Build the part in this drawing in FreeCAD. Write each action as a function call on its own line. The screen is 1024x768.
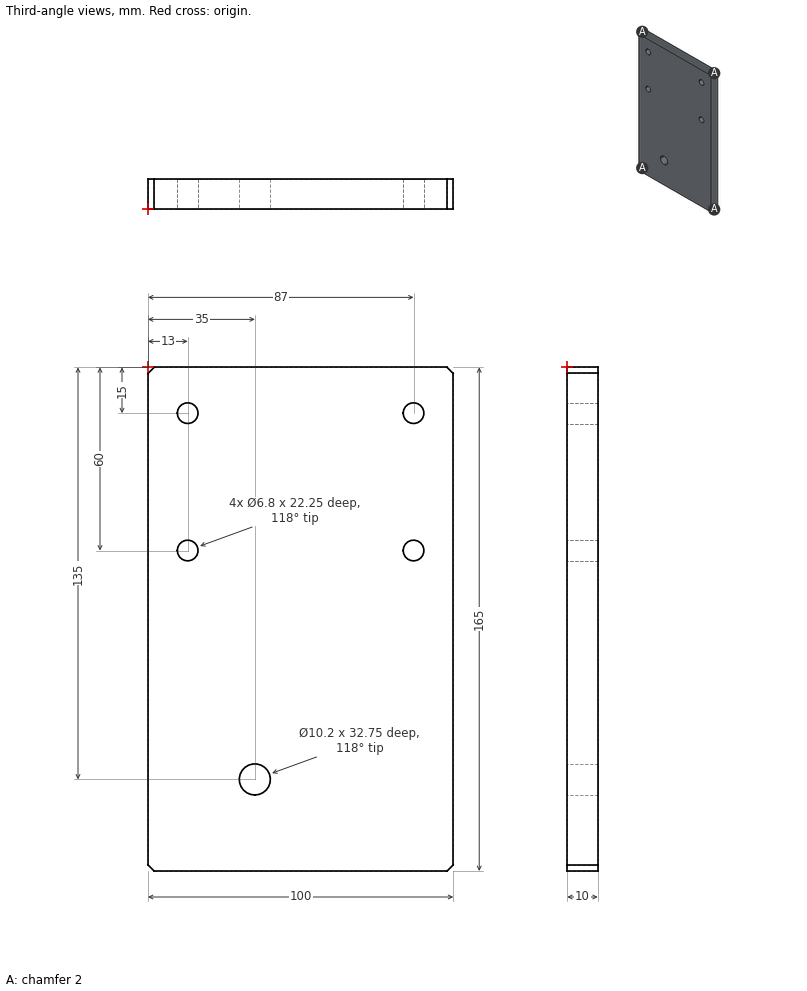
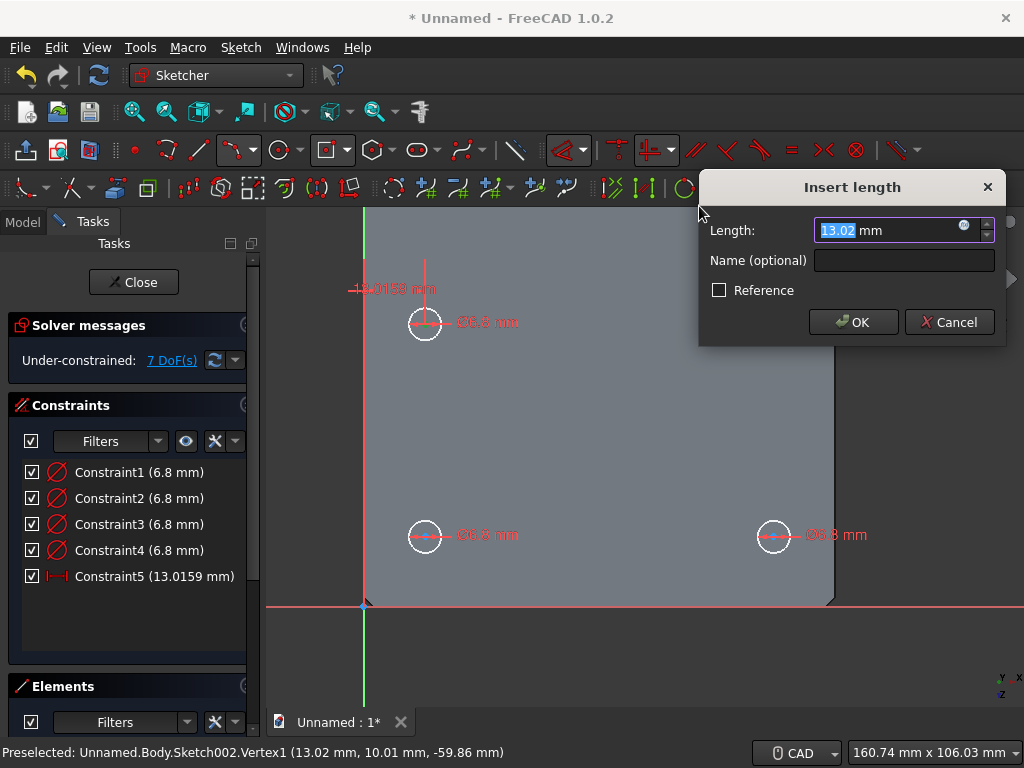
text(13)
key(Return)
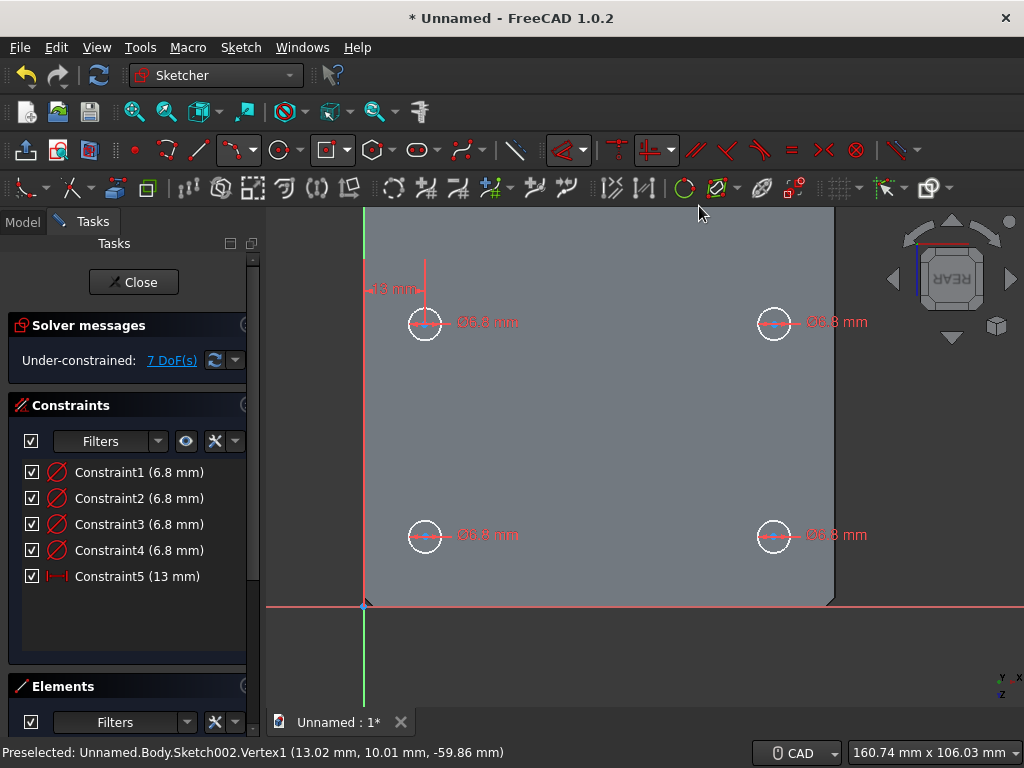
click(425, 324)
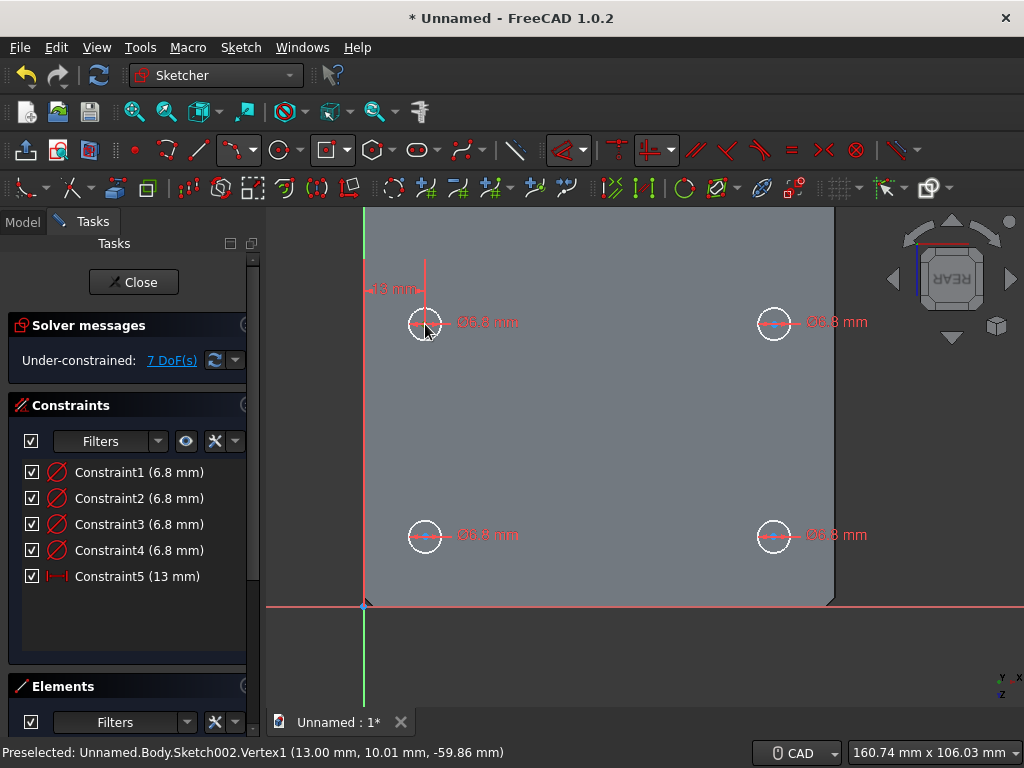
key(i)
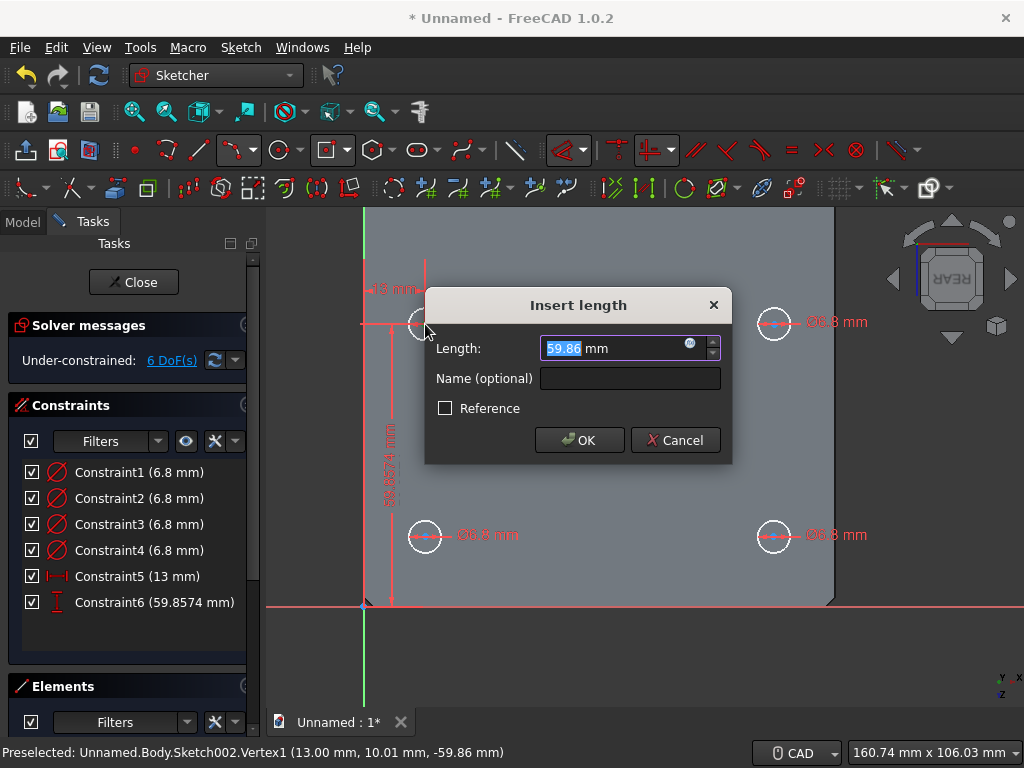
text(60)
key(Return)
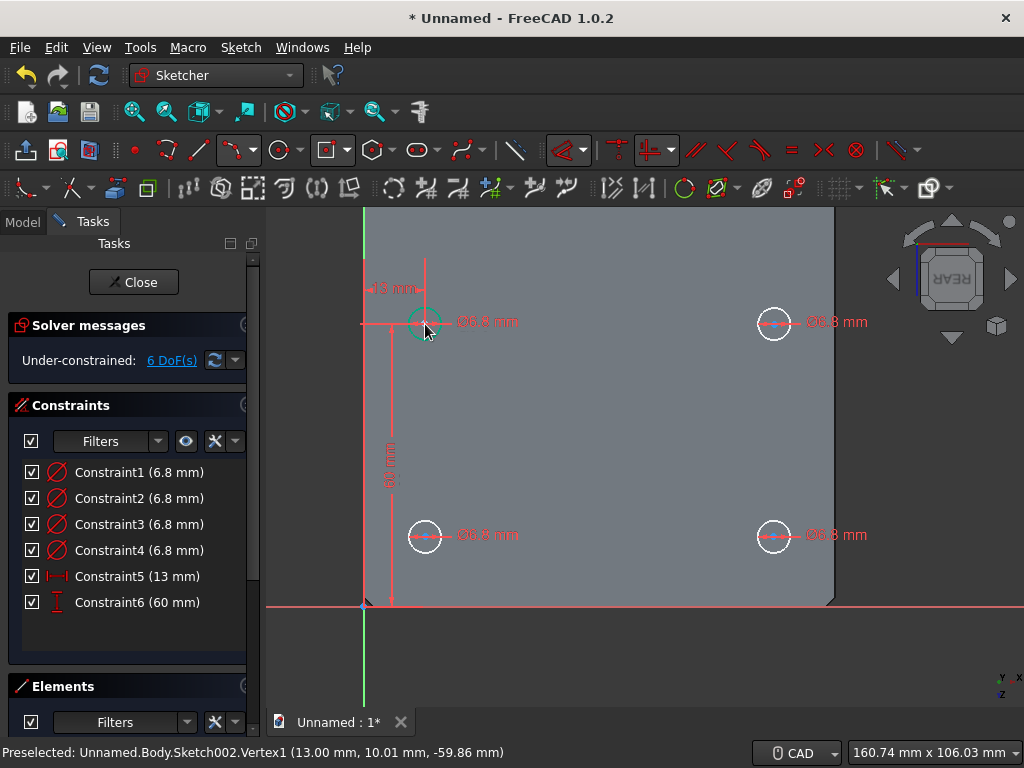
click(425, 537)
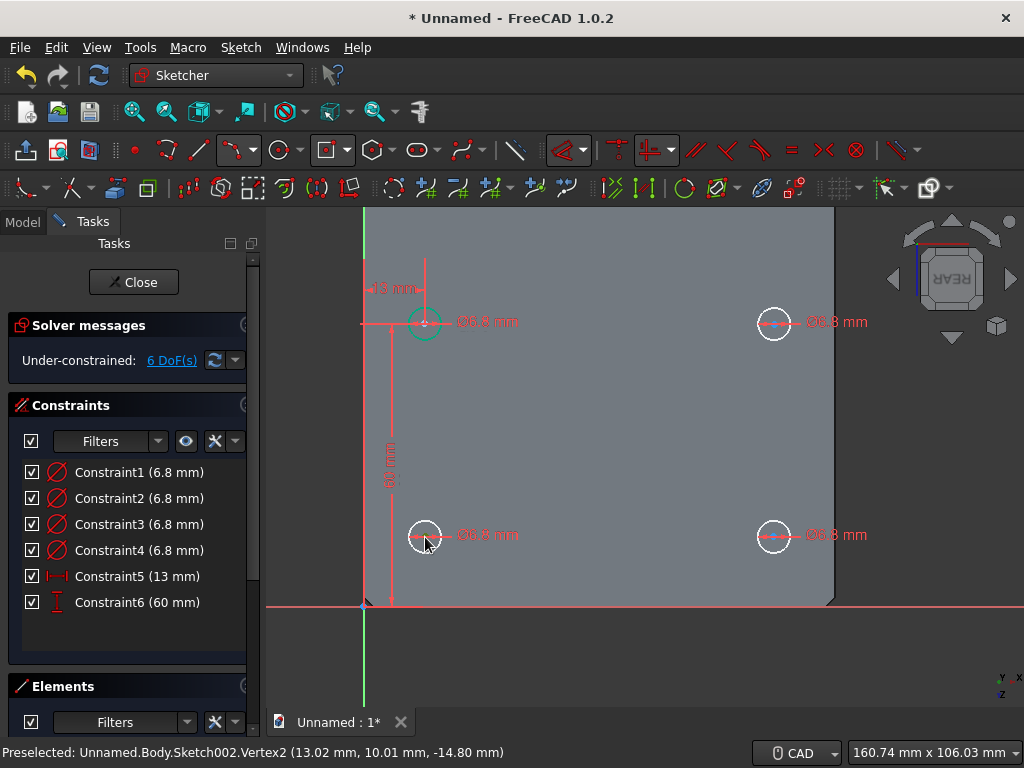
key(l)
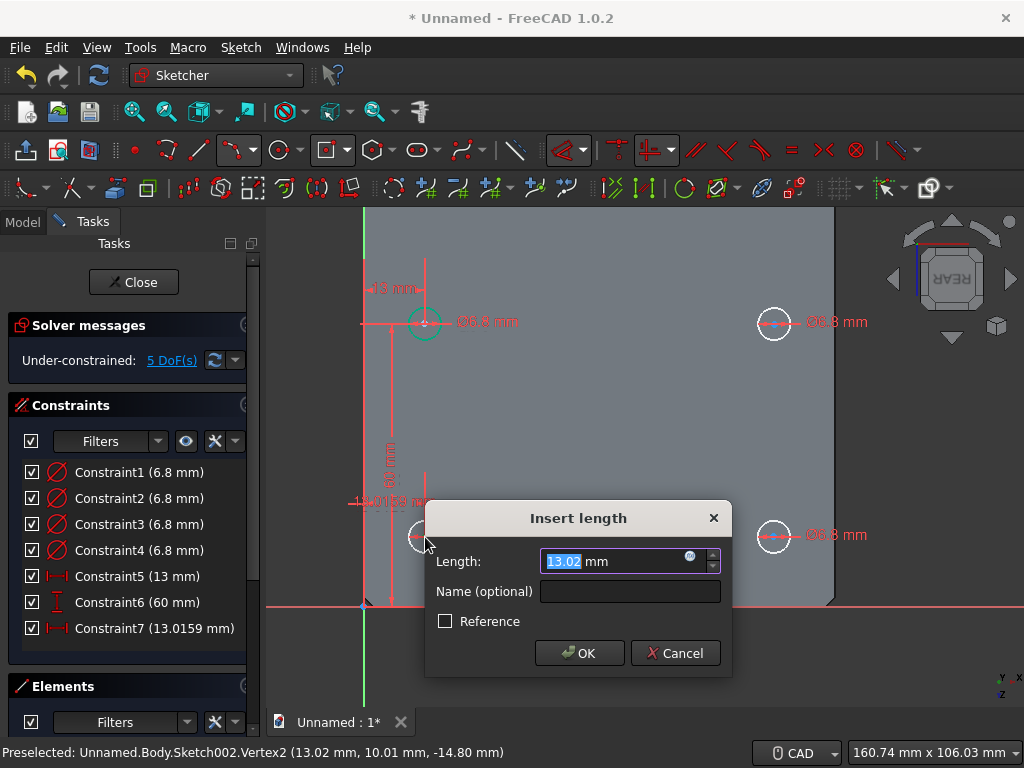
text(13)
key(Return)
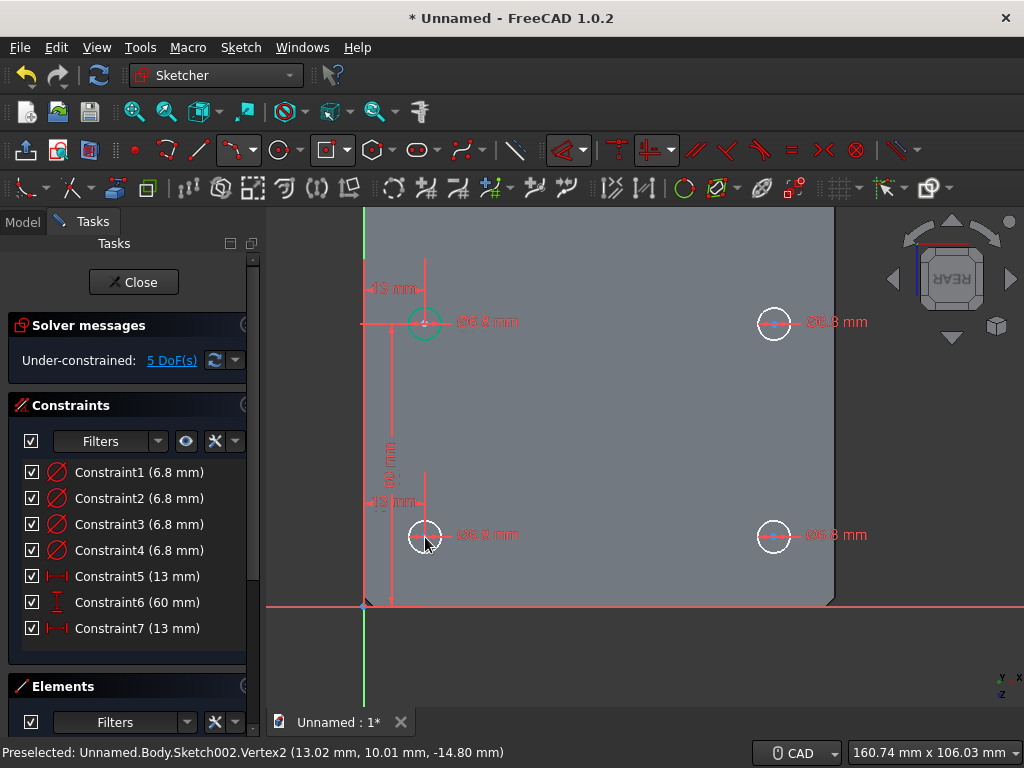
click(425, 537)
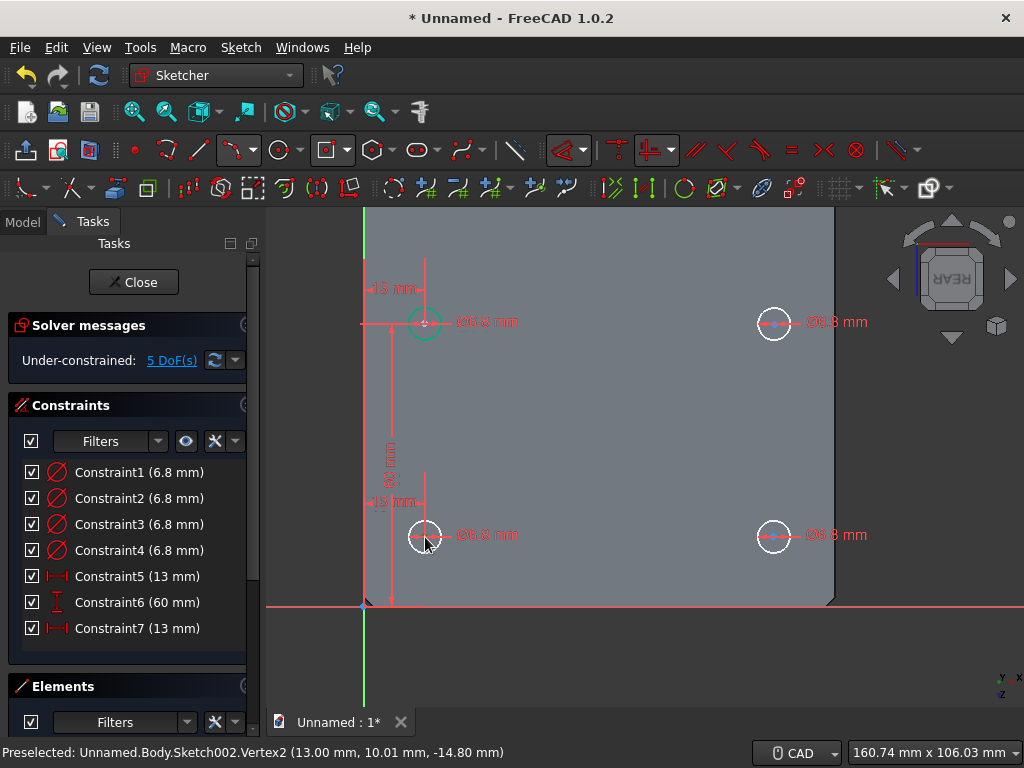
click(586, 150)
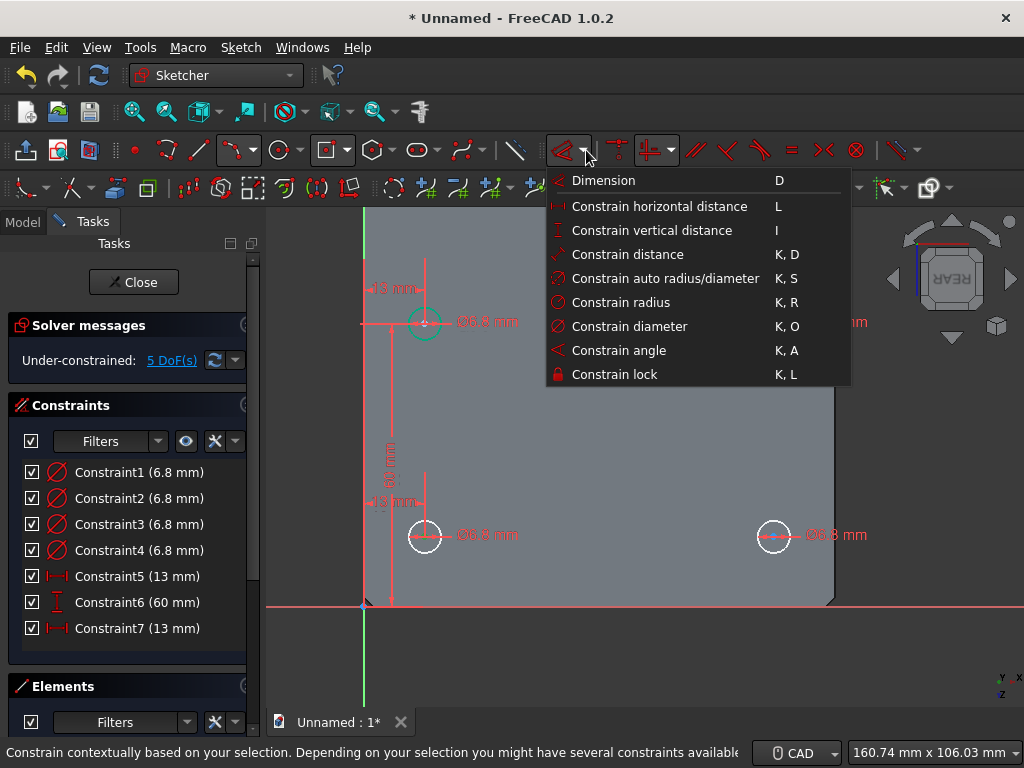
click(699, 230)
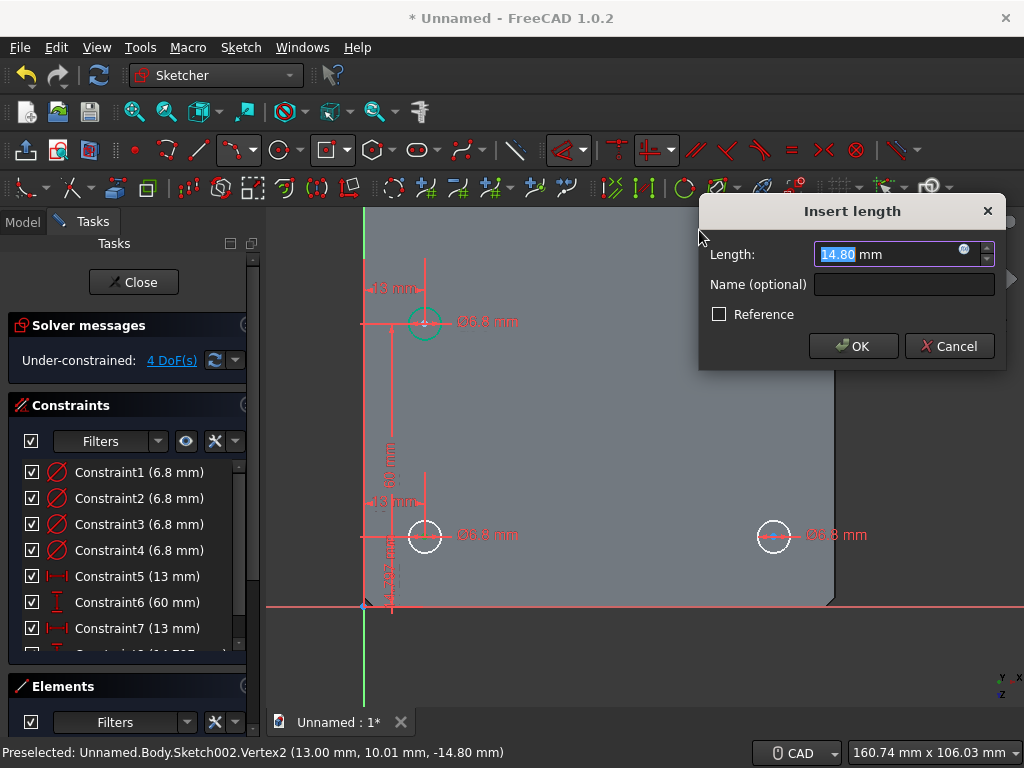
text(15)
key(Return)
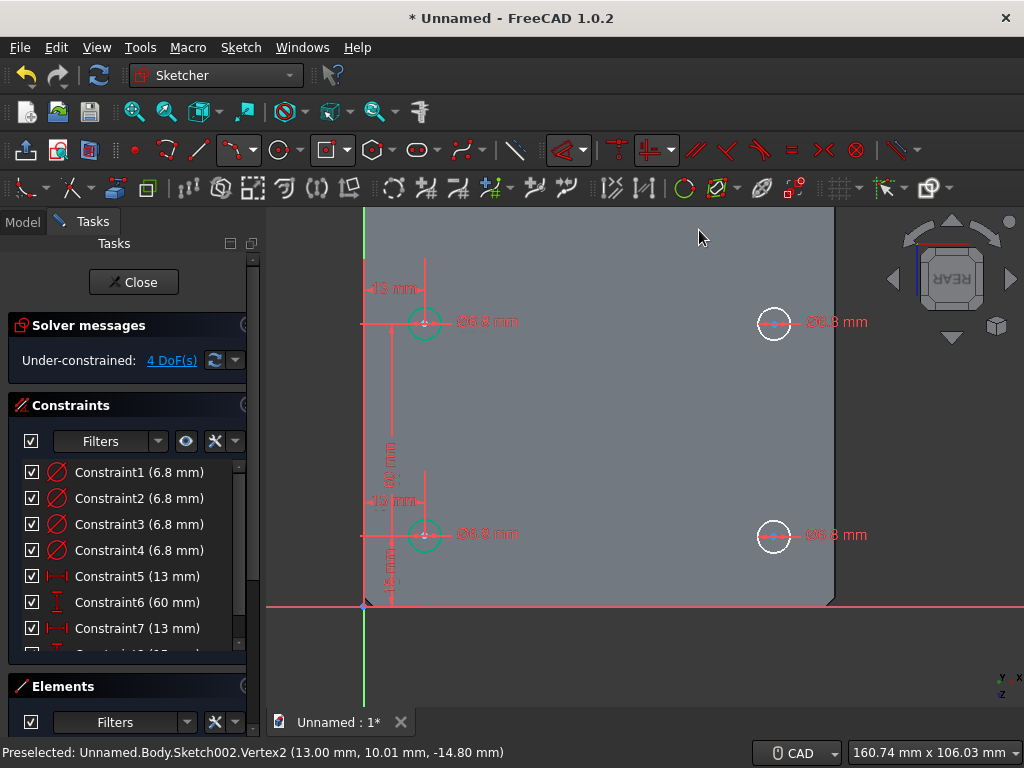
click(774, 537)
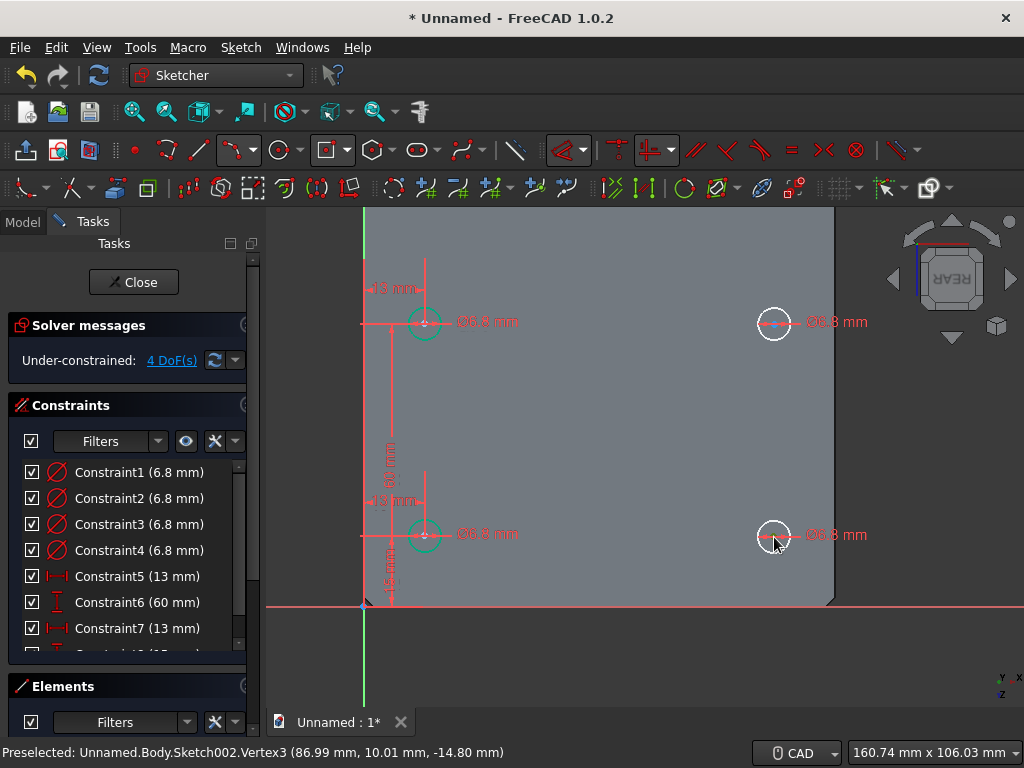
click(586, 150)